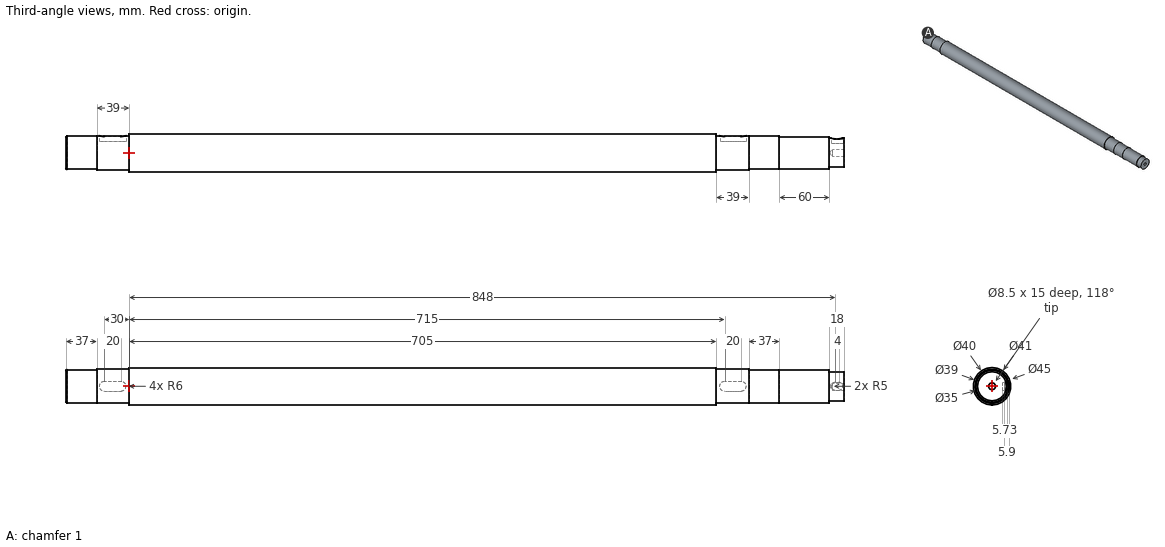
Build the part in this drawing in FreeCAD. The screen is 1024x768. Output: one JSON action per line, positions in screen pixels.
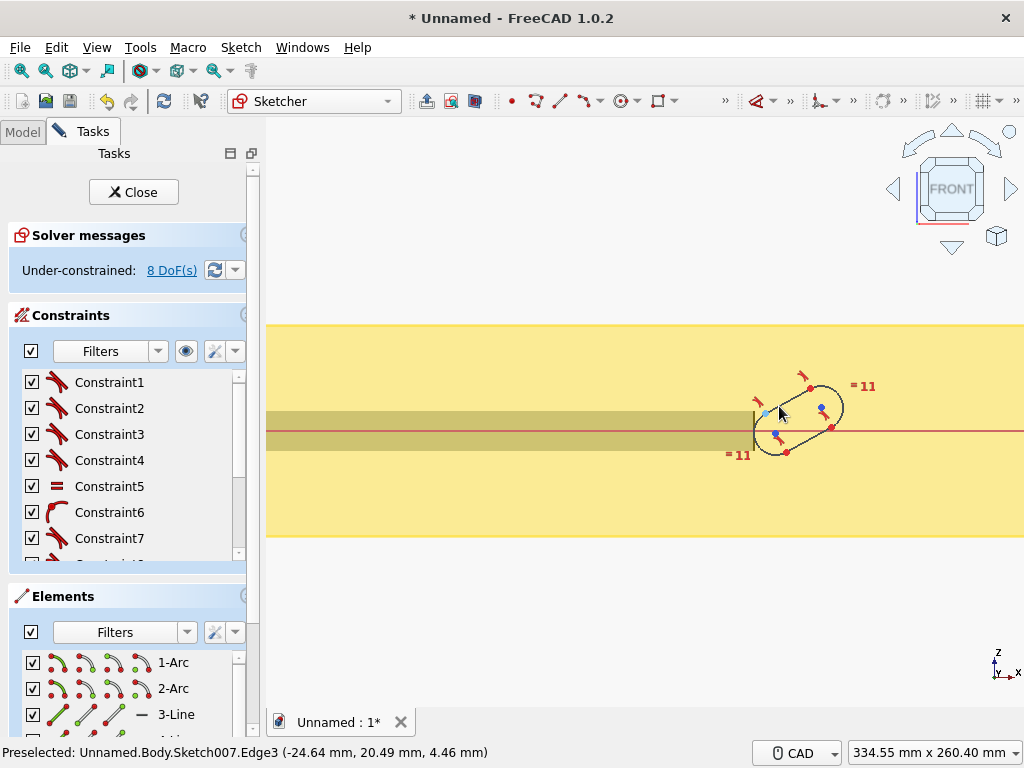
{"action": "left_click", "coordinate": [779, 406]}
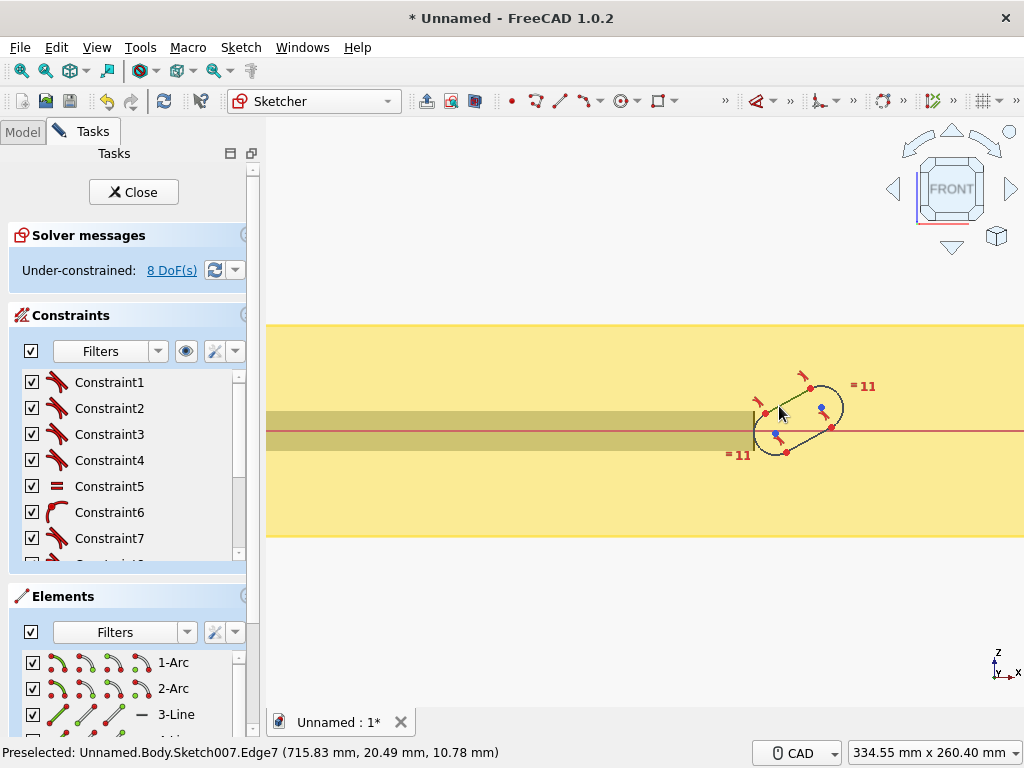
{"action": "key", "text": "h"}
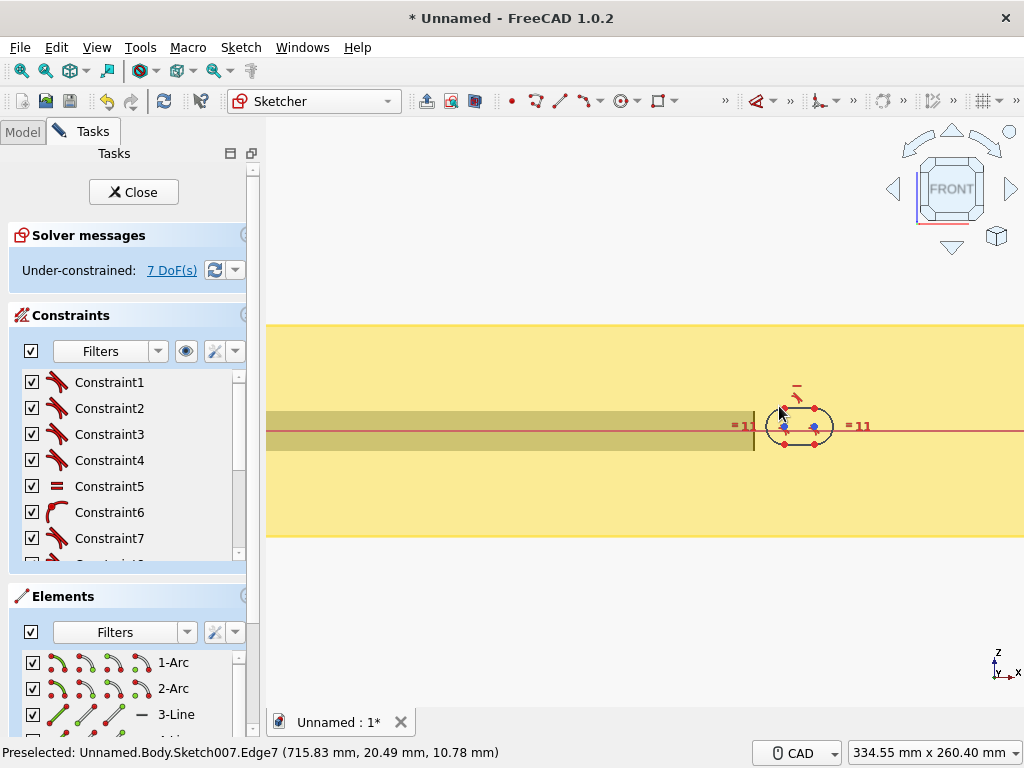
{"action": "scroll", "coordinate": [780, 406], "scroll_direction": "down", "scroll_amount": 7}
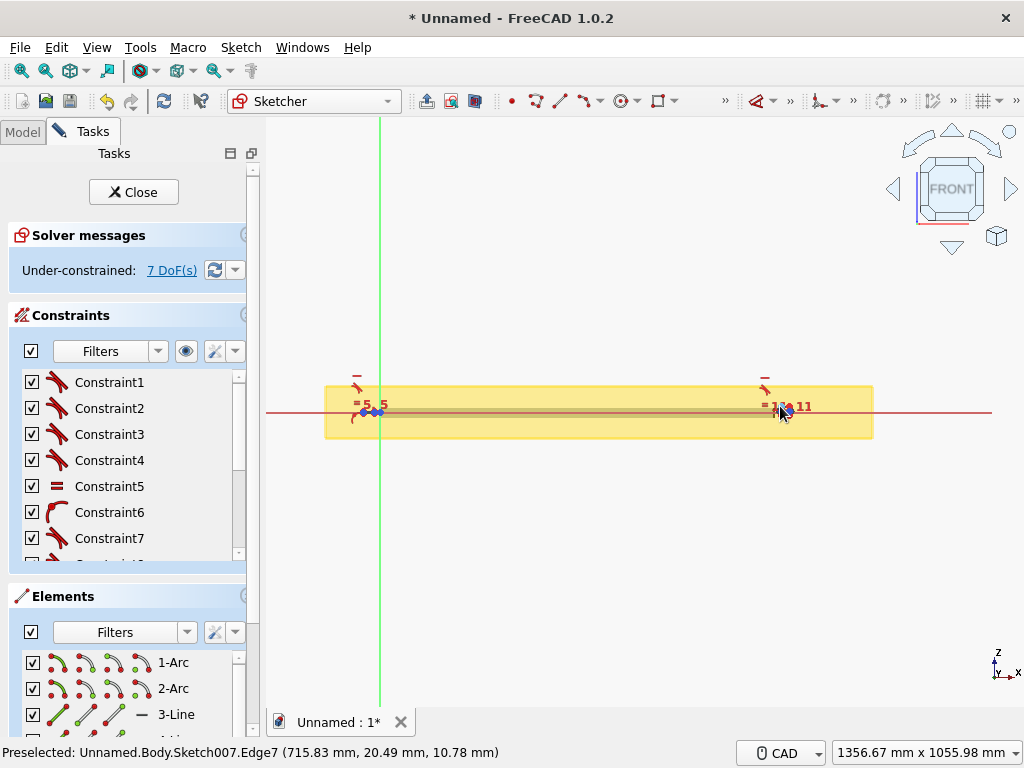
{"action": "scroll", "coordinate": [363, 413], "scroll_direction": "up", "scroll_amount": 14}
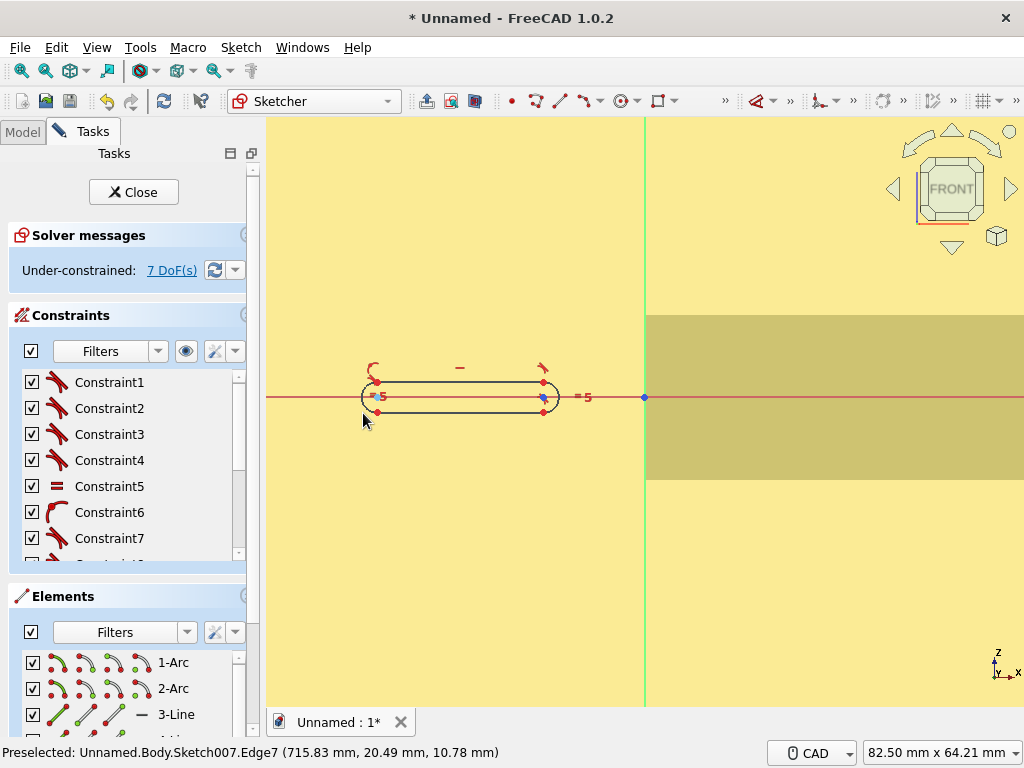
{"action": "left_click", "coordinate": [362, 397]}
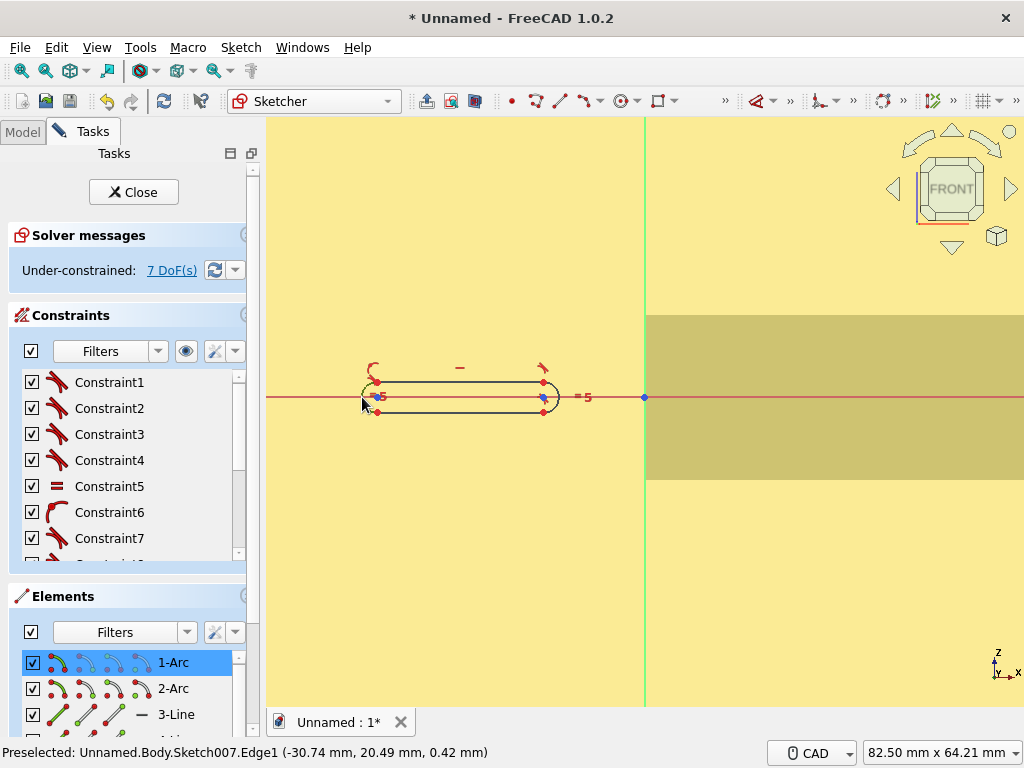
{"action": "scroll", "coordinate": [362, 413], "scroll_direction": "down", "scroll_amount": 14}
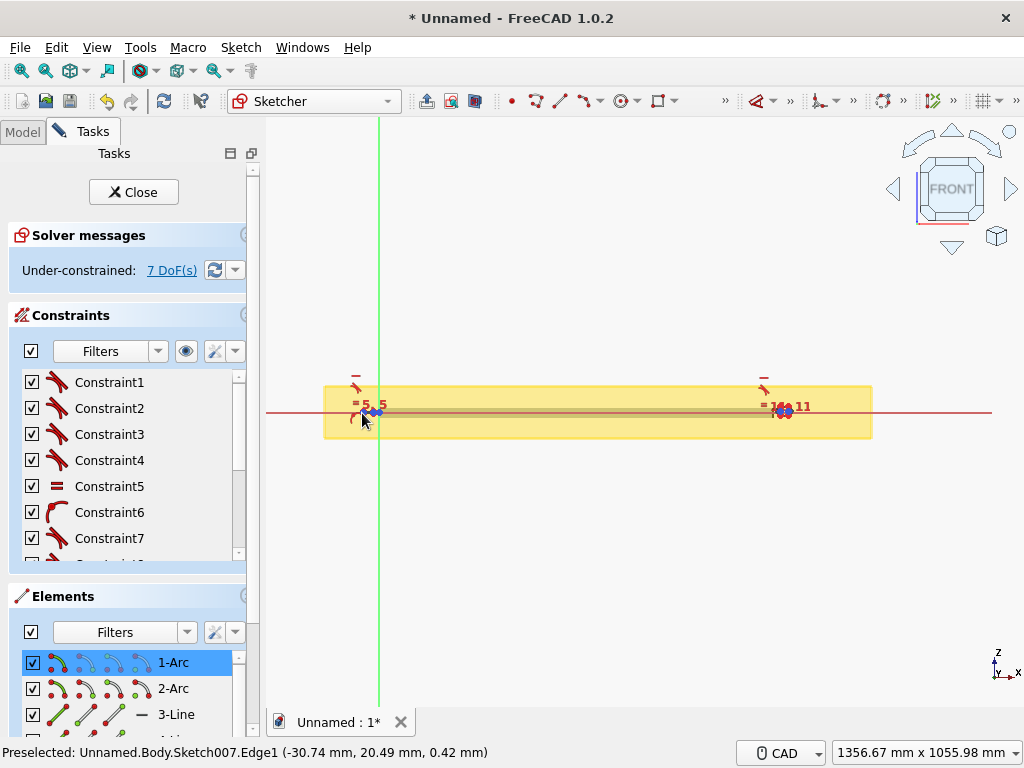
{"action": "scroll", "coordinate": [777, 409], "scroll_direction": "up", "scroll_amount": 7}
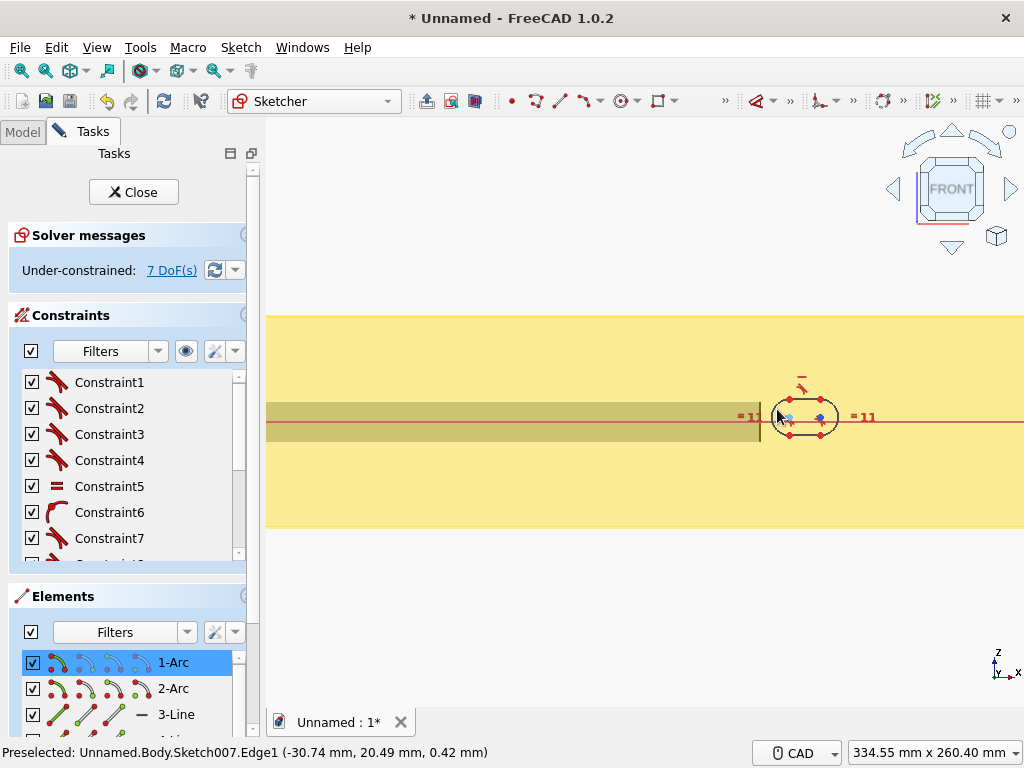
{"action": "left_click", "coordinate": [775, 407]}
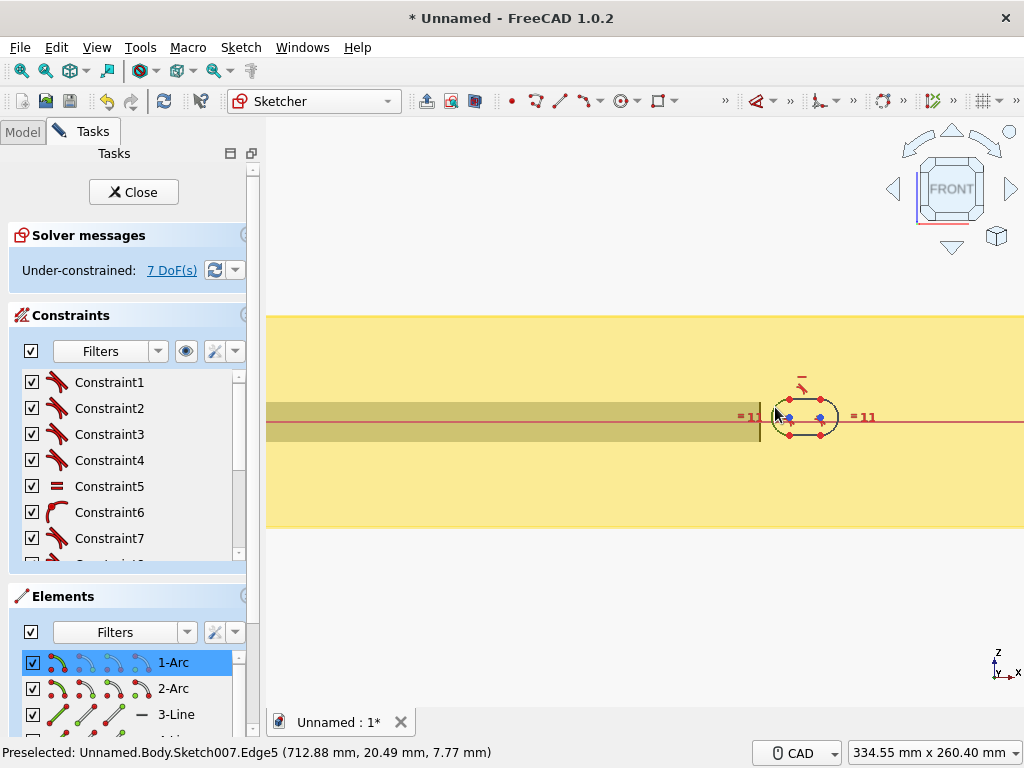
{"action": "key", "text": "e"}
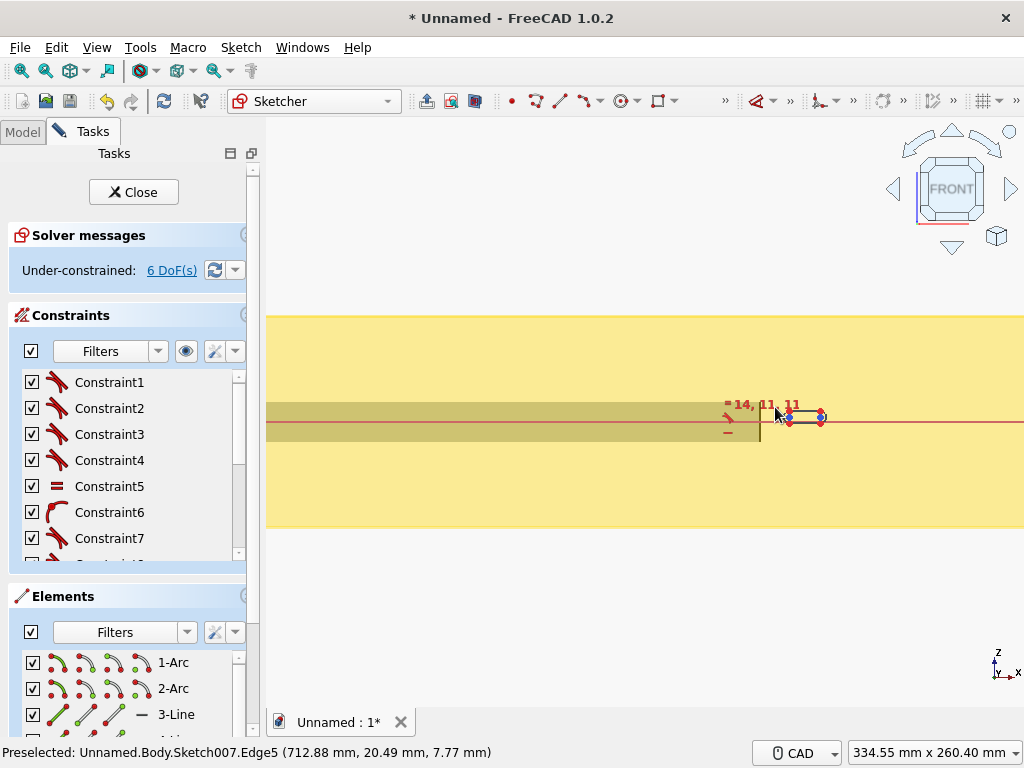
{"action": "scroll", "coordinate": [790, 417], "scroll_direction": "up", "scroll_amount": 4}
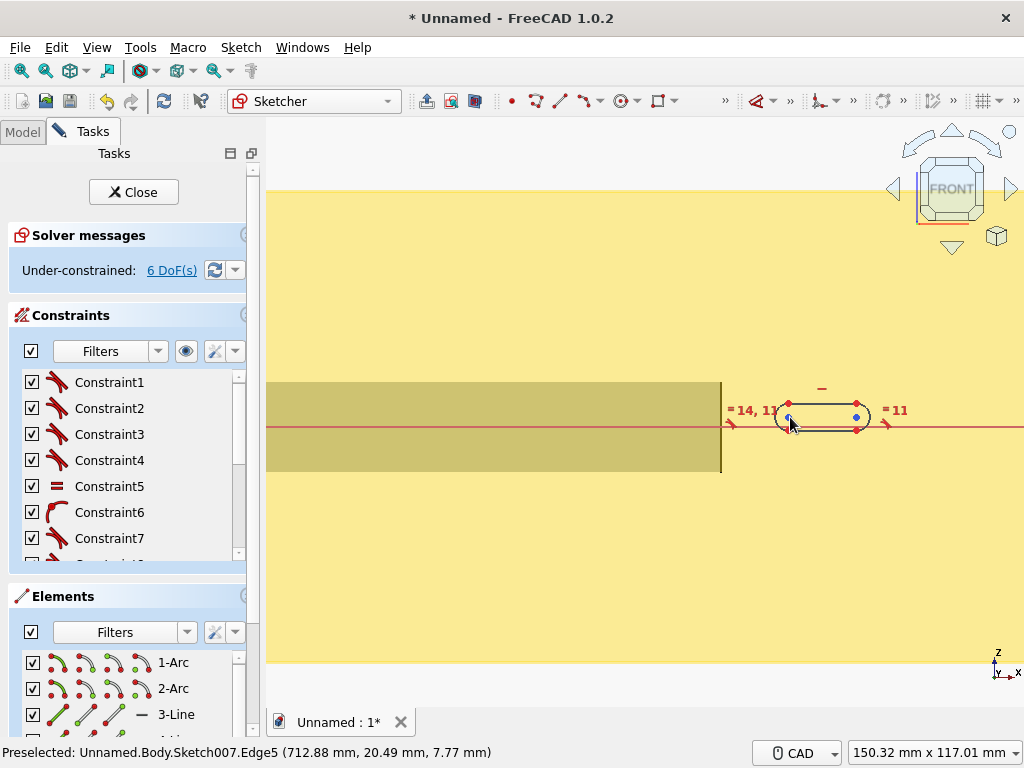
{"action": "left_click", "coordinate": [789, 417]}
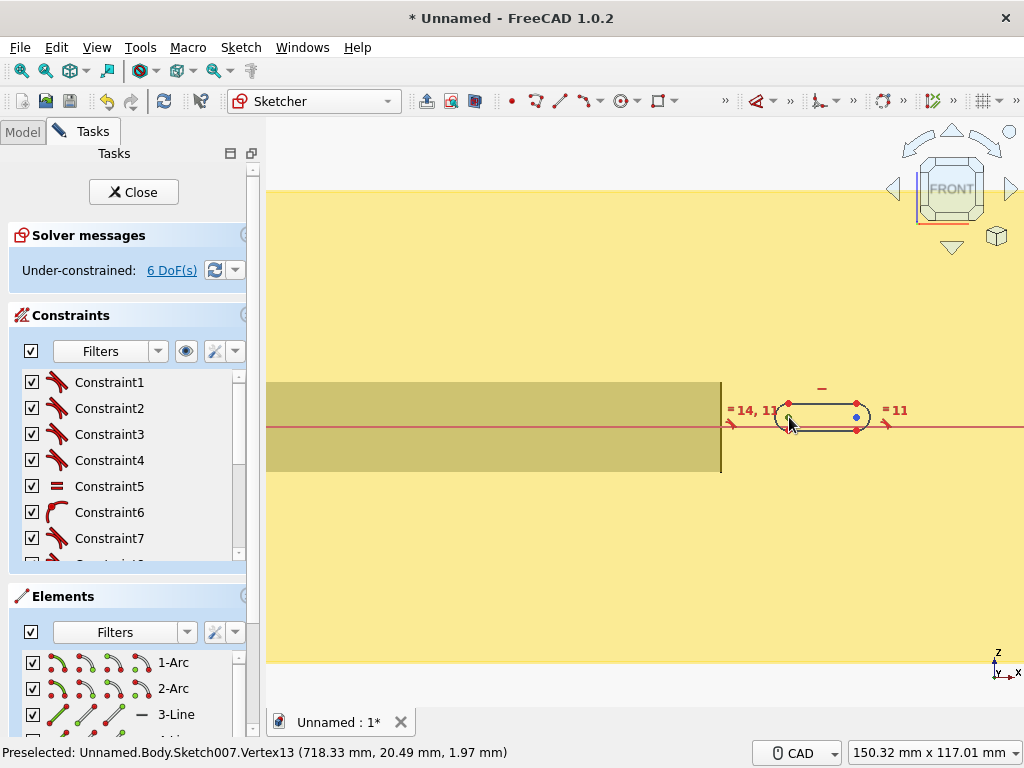
{"action": "left_click", "coordinate": [334, 427]}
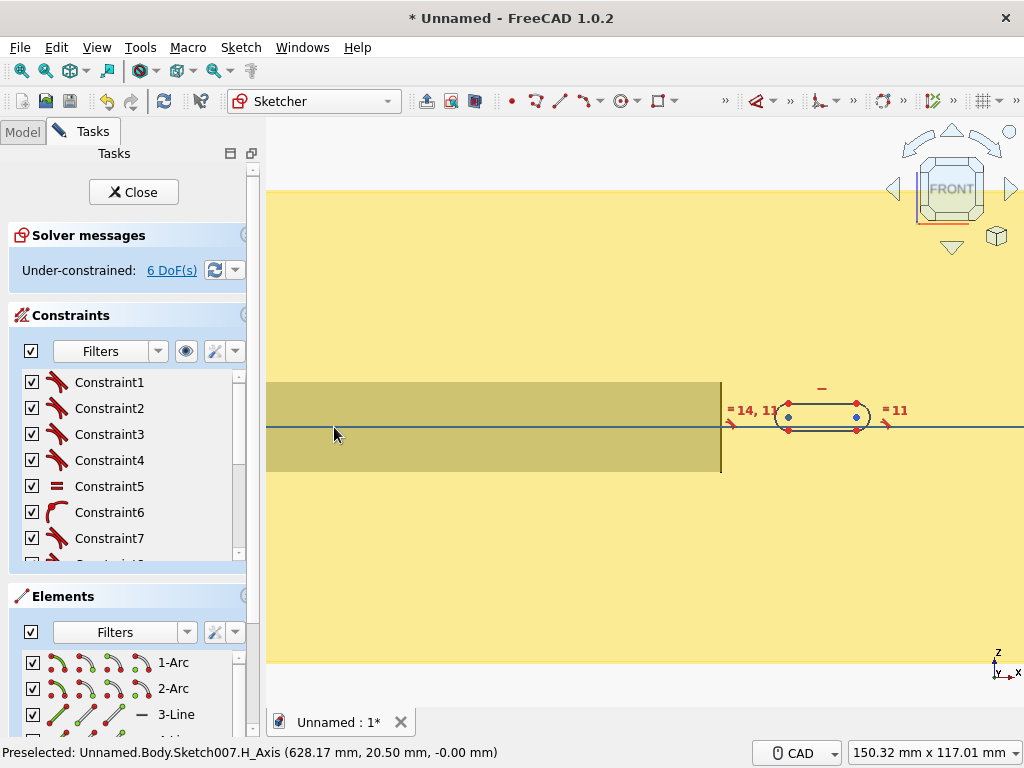
{"action": "key", "text": "c"}